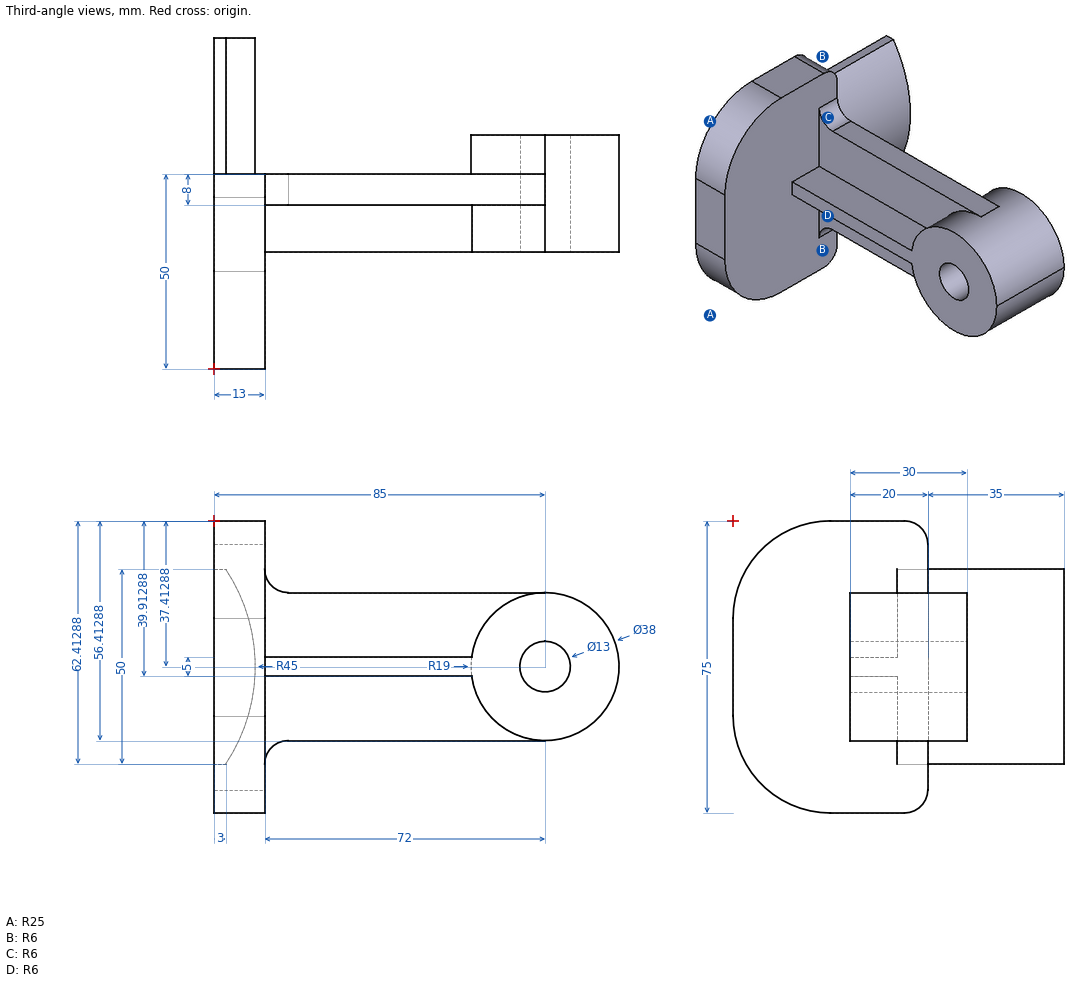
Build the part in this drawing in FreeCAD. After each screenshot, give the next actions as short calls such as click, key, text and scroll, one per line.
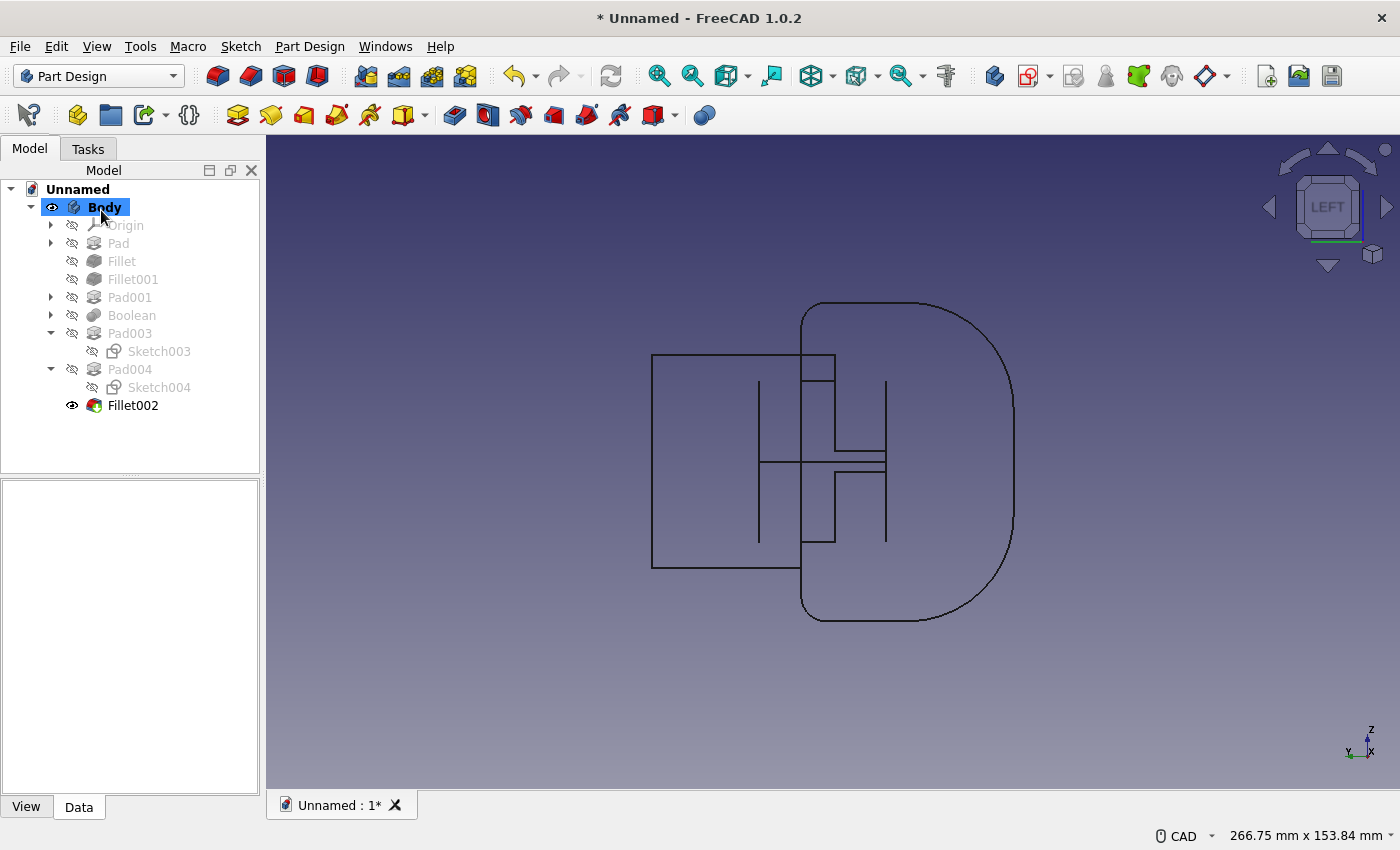
key(0)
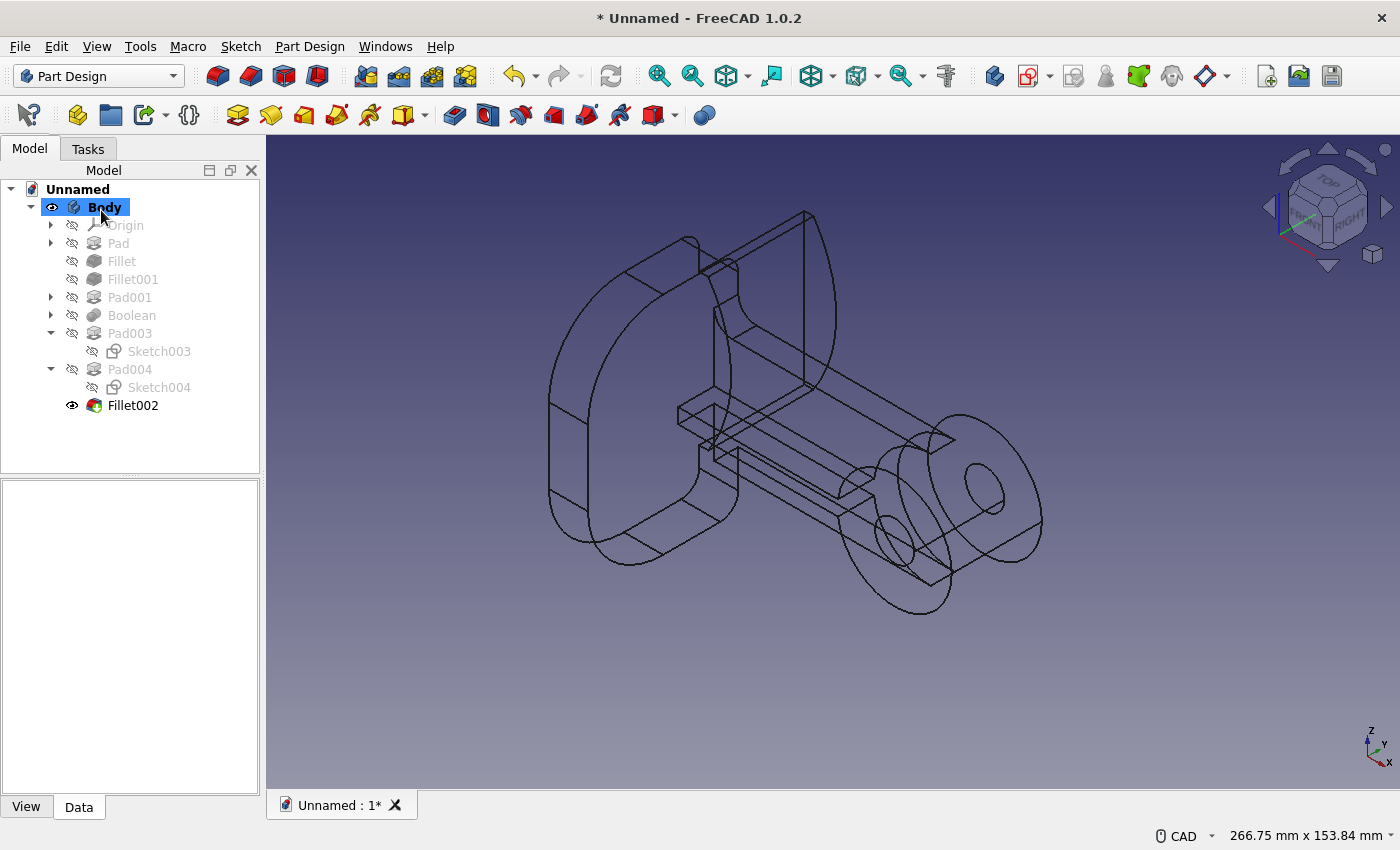
click(721, 456)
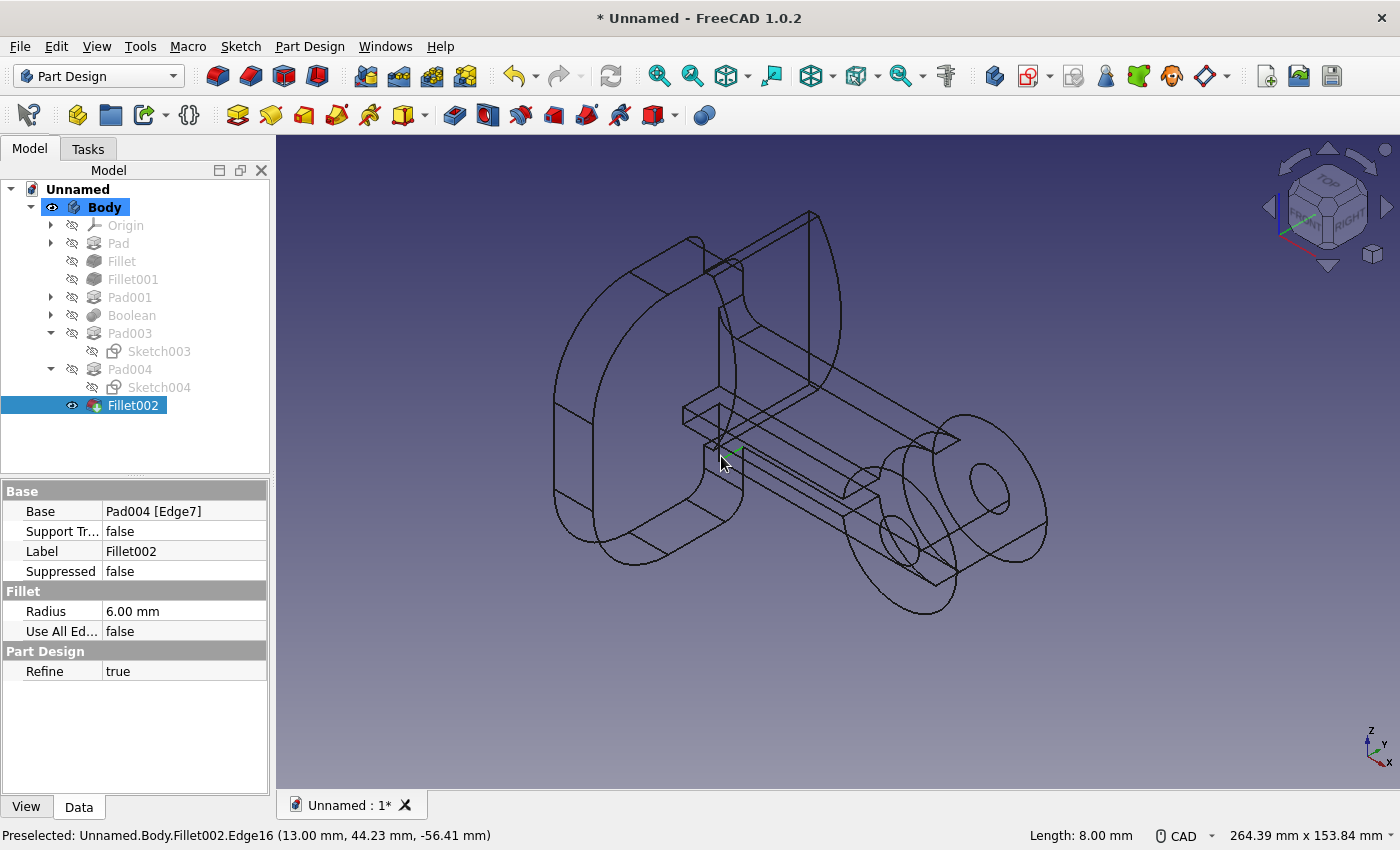
key(v)
key(1)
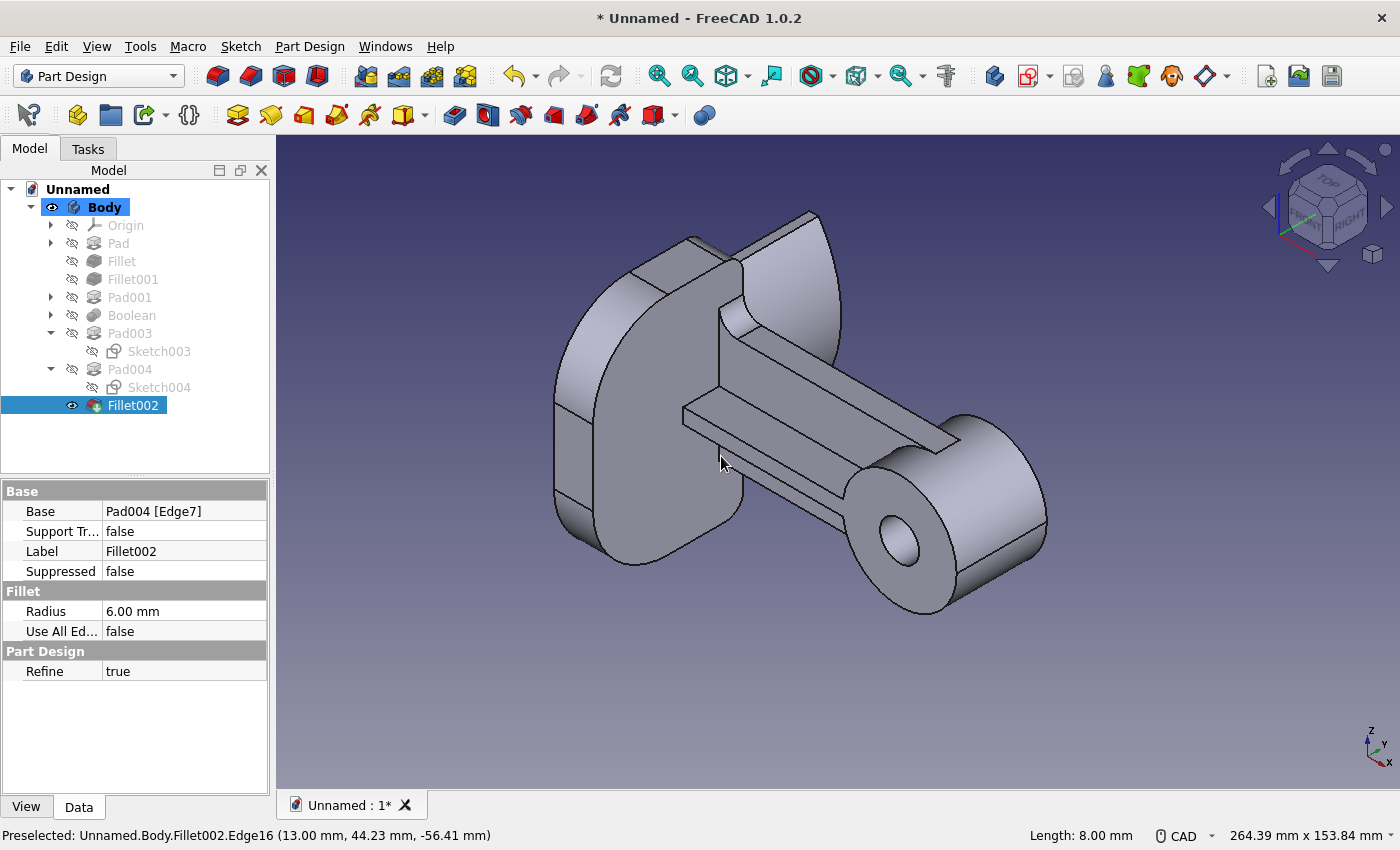
click(218, 76)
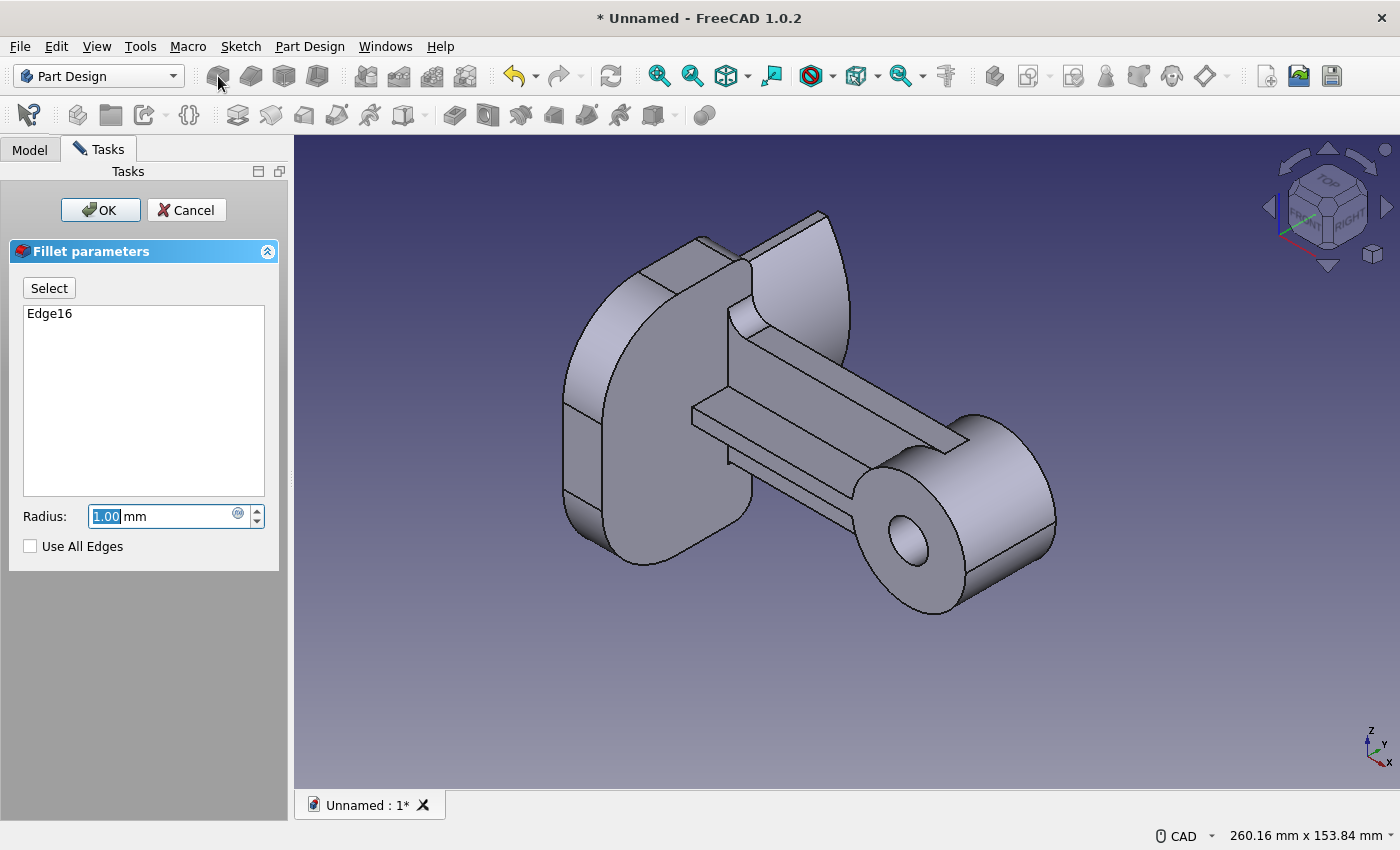
text(6)
key(Tab)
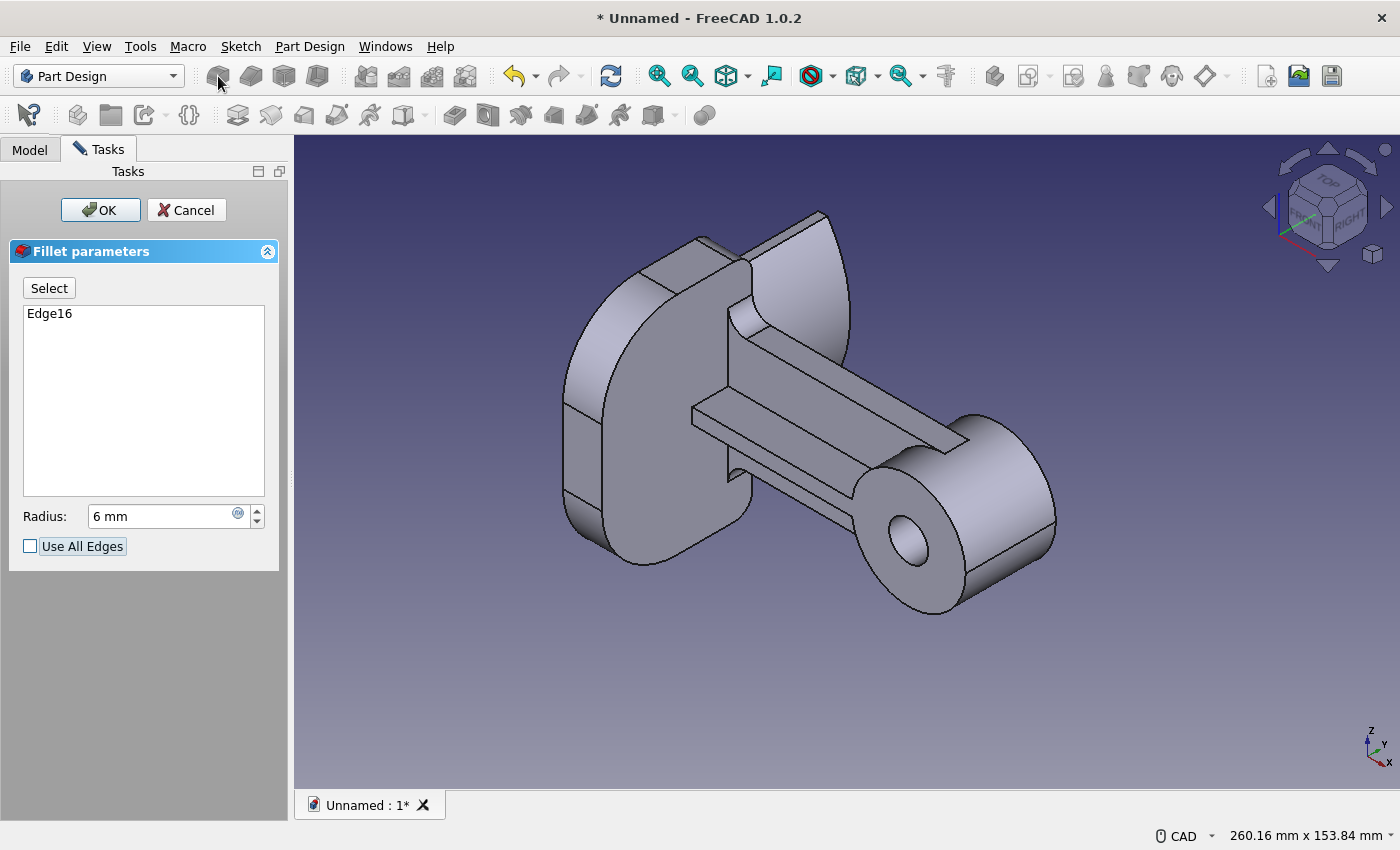
click(101, 210)